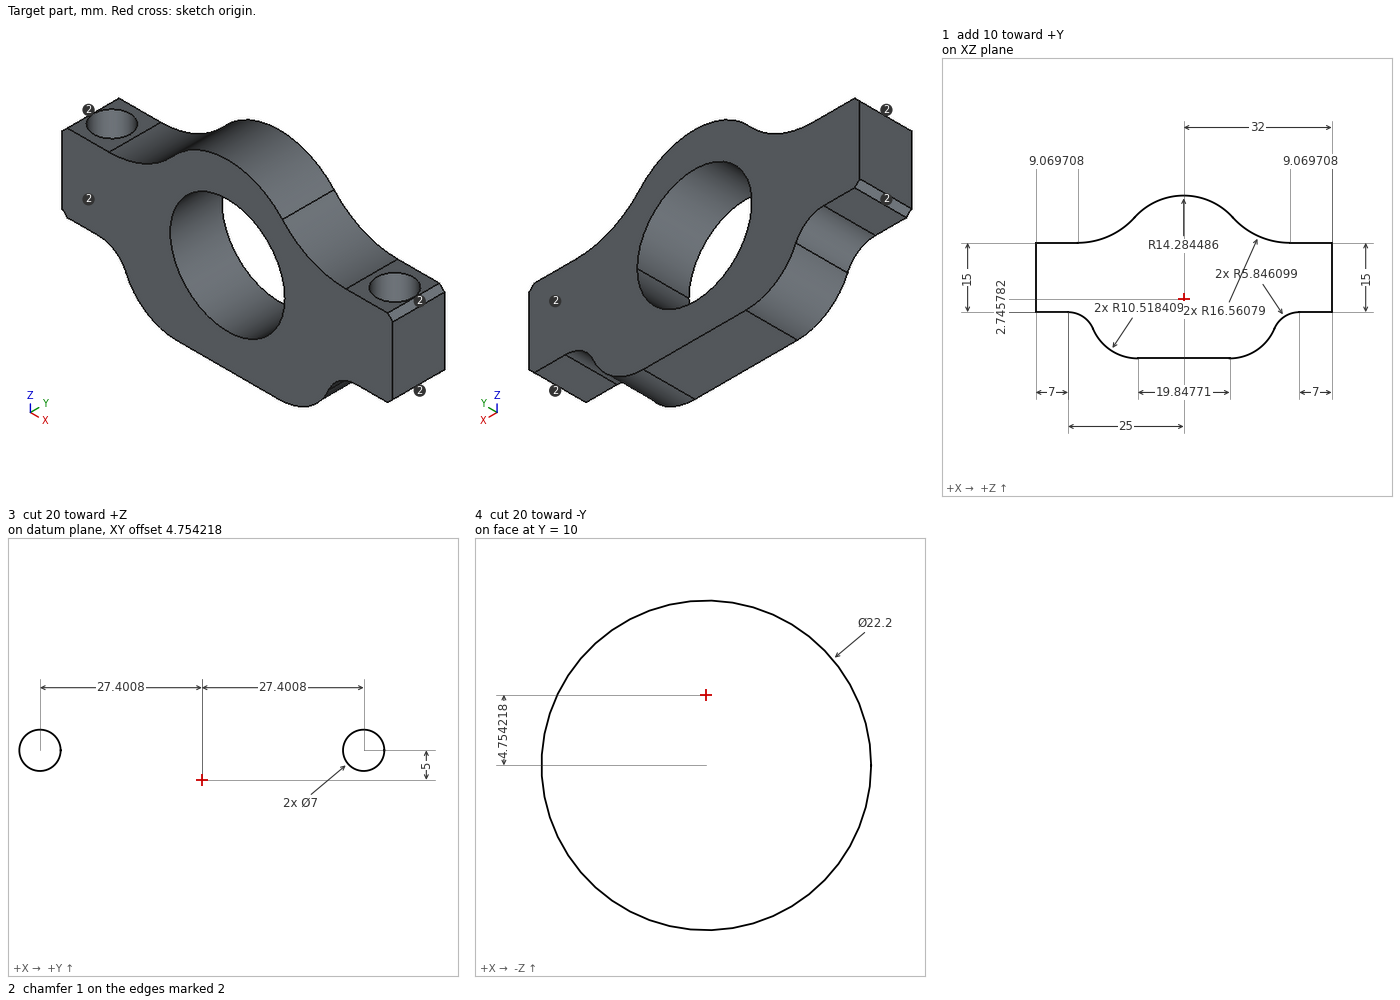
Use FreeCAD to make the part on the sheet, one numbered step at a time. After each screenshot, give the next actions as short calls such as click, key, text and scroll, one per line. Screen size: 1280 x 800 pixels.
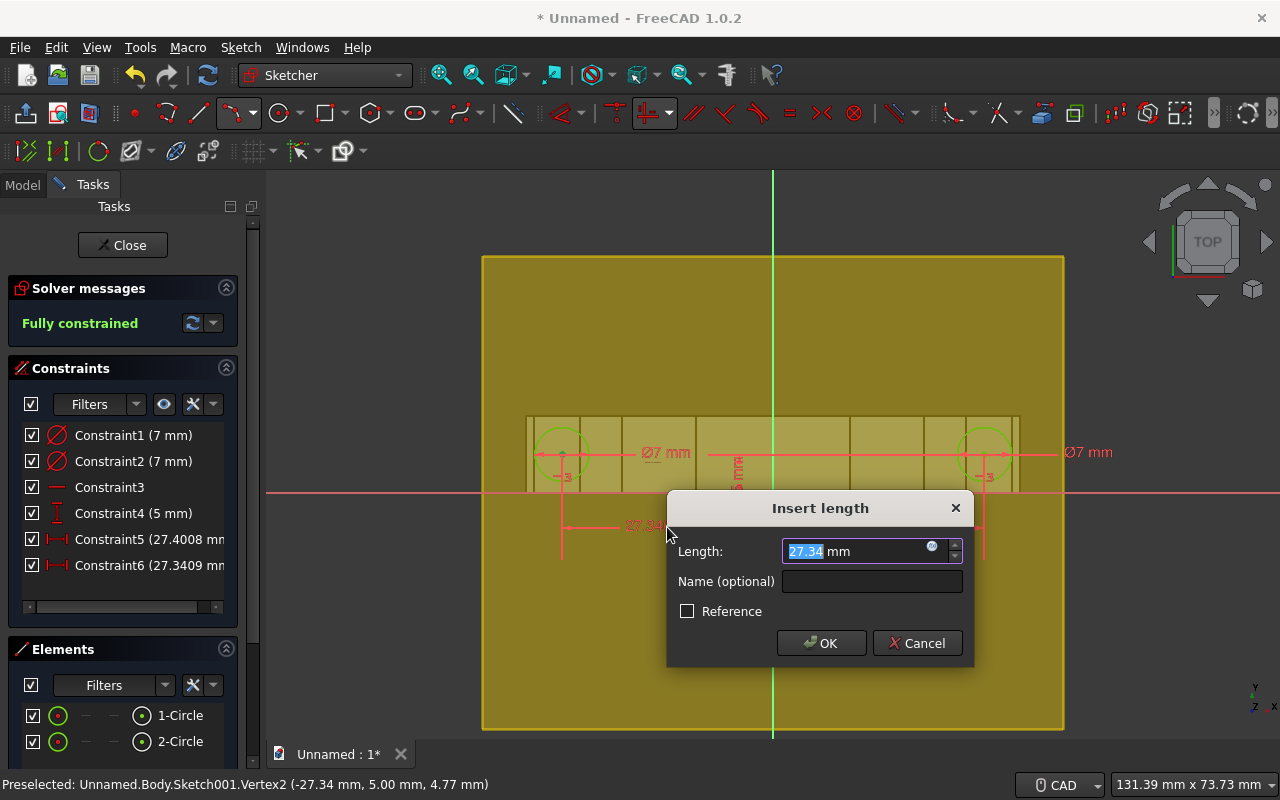
text(27.4008)
key(Return)
key(Escape)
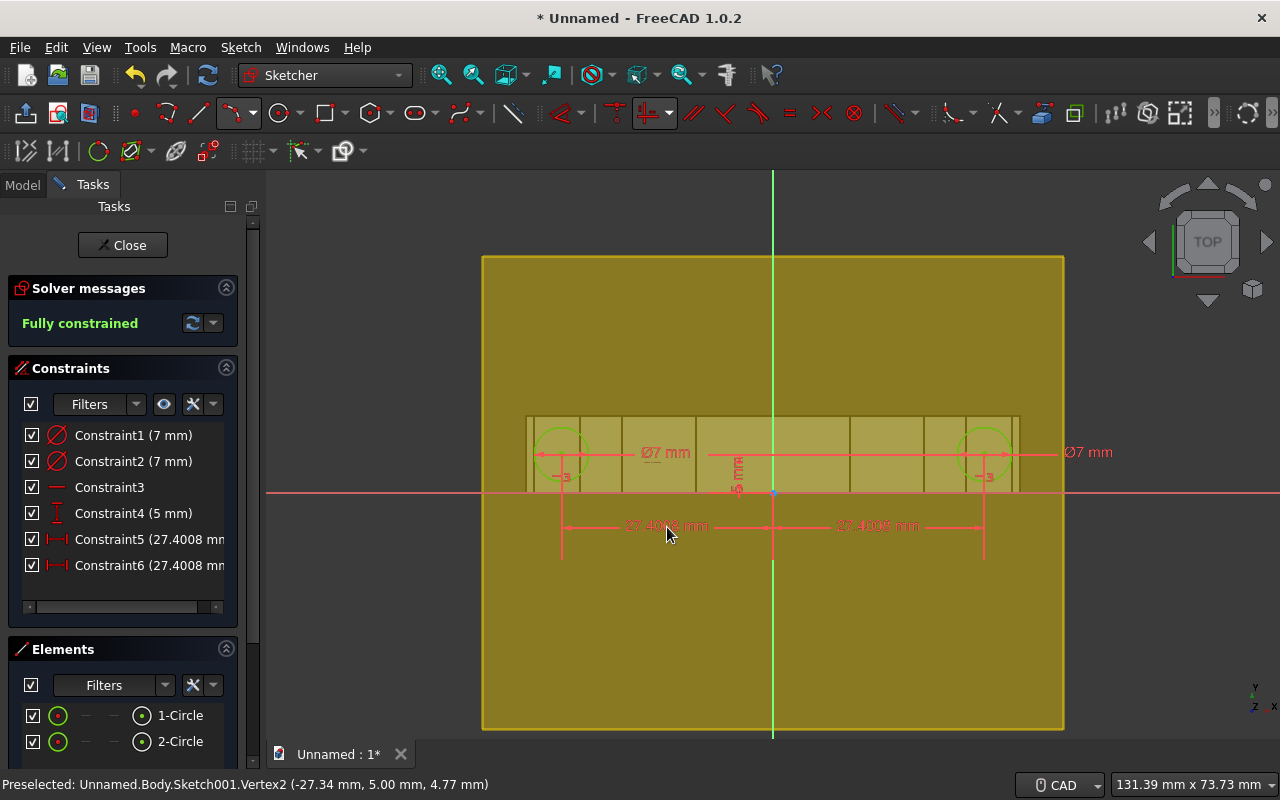
click(123, 245)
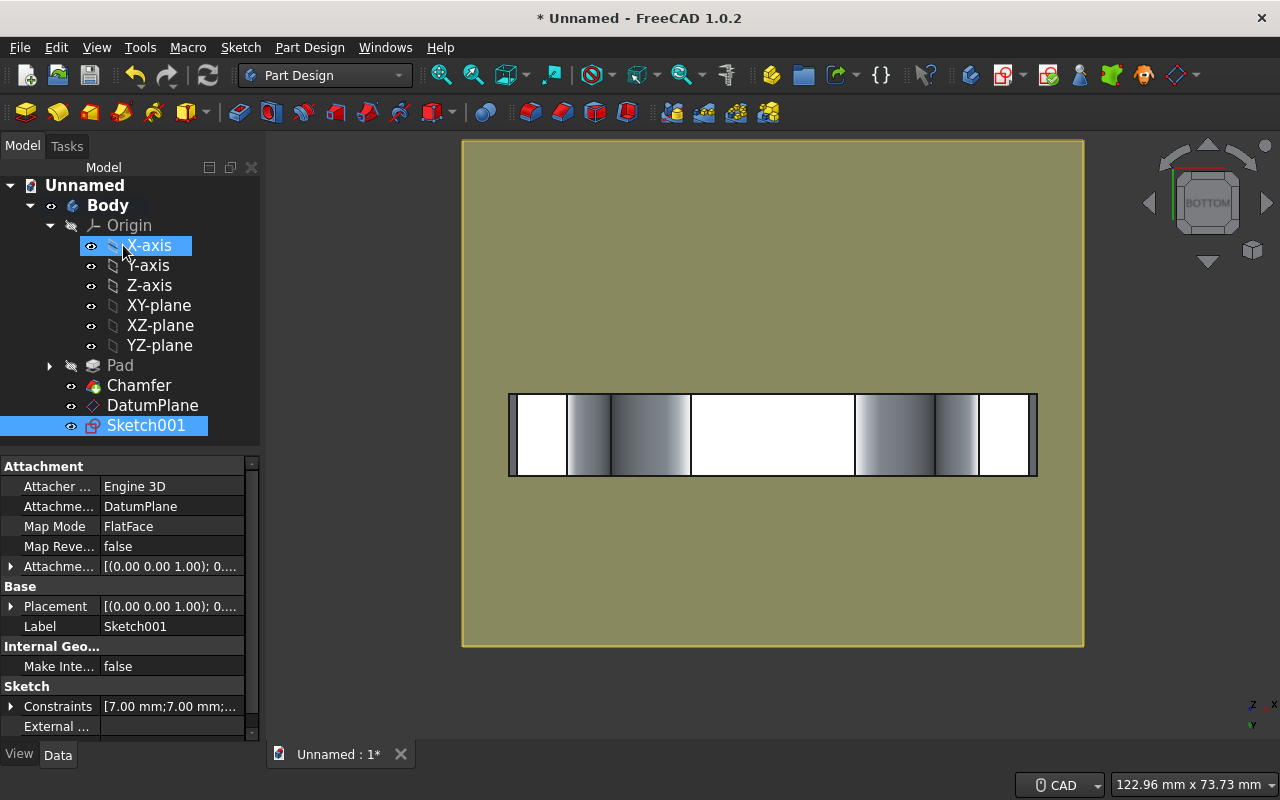
click(240, 112)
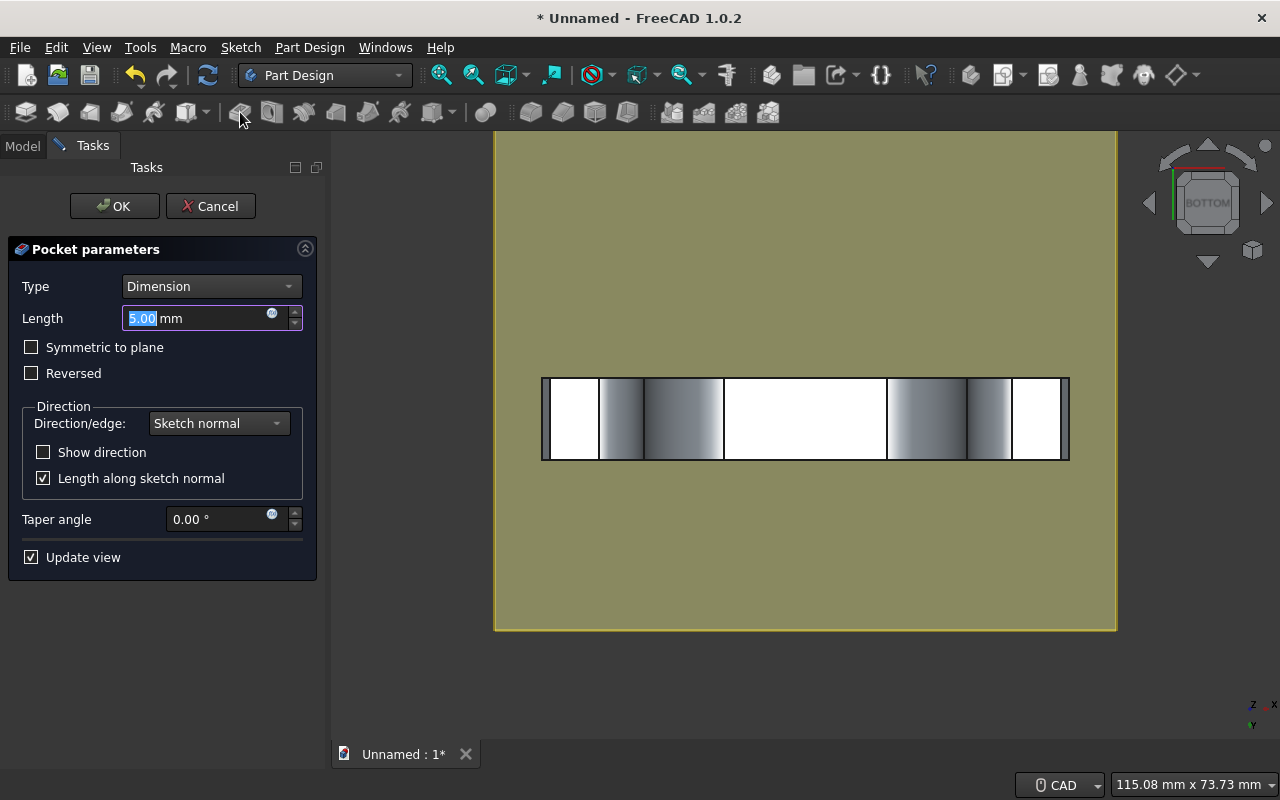
text(20)
key(Tab)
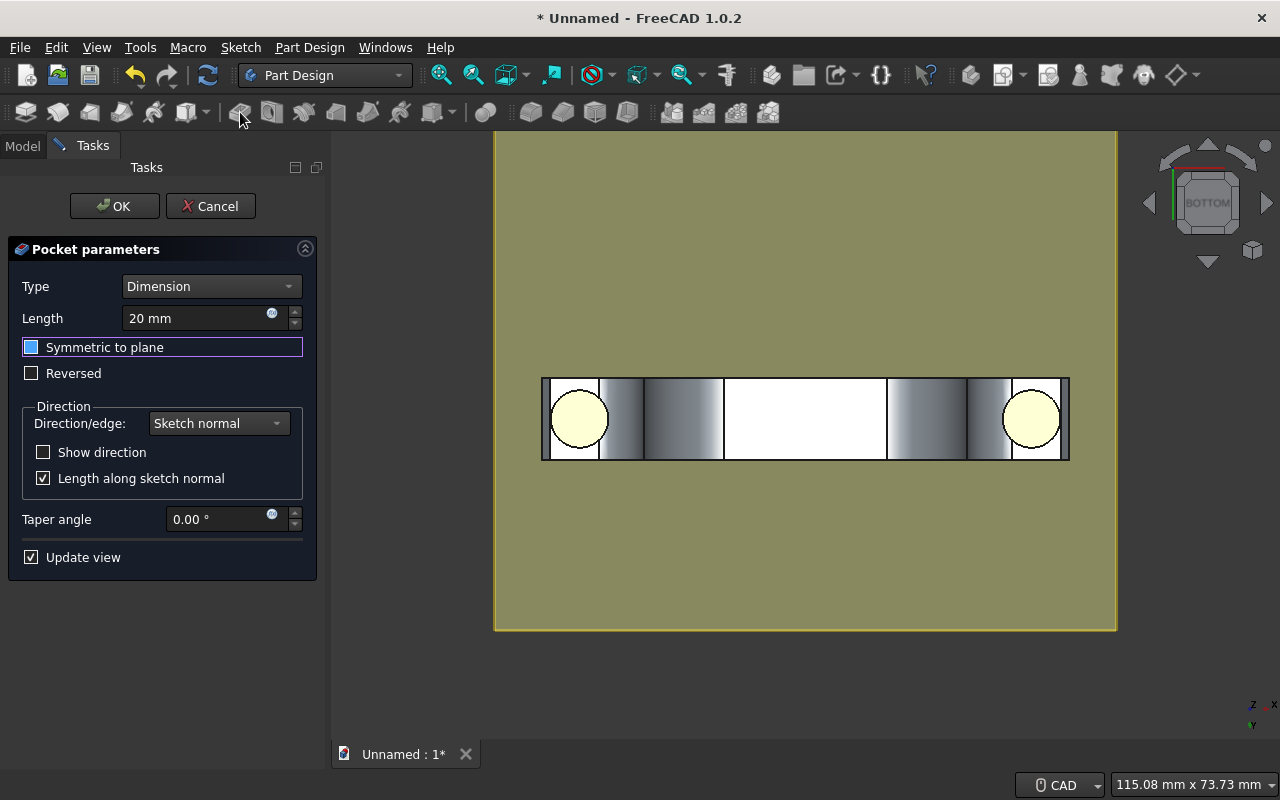
click(30, 373)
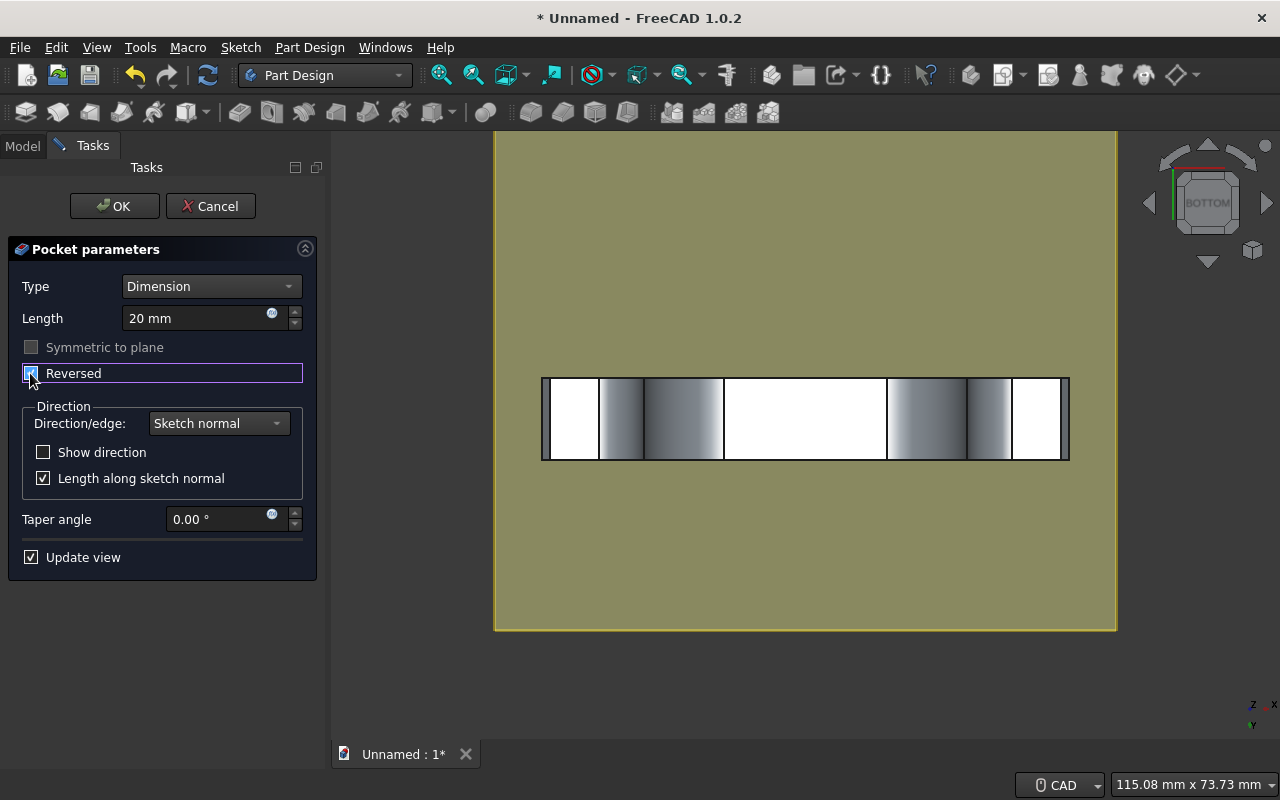
click(115, 206)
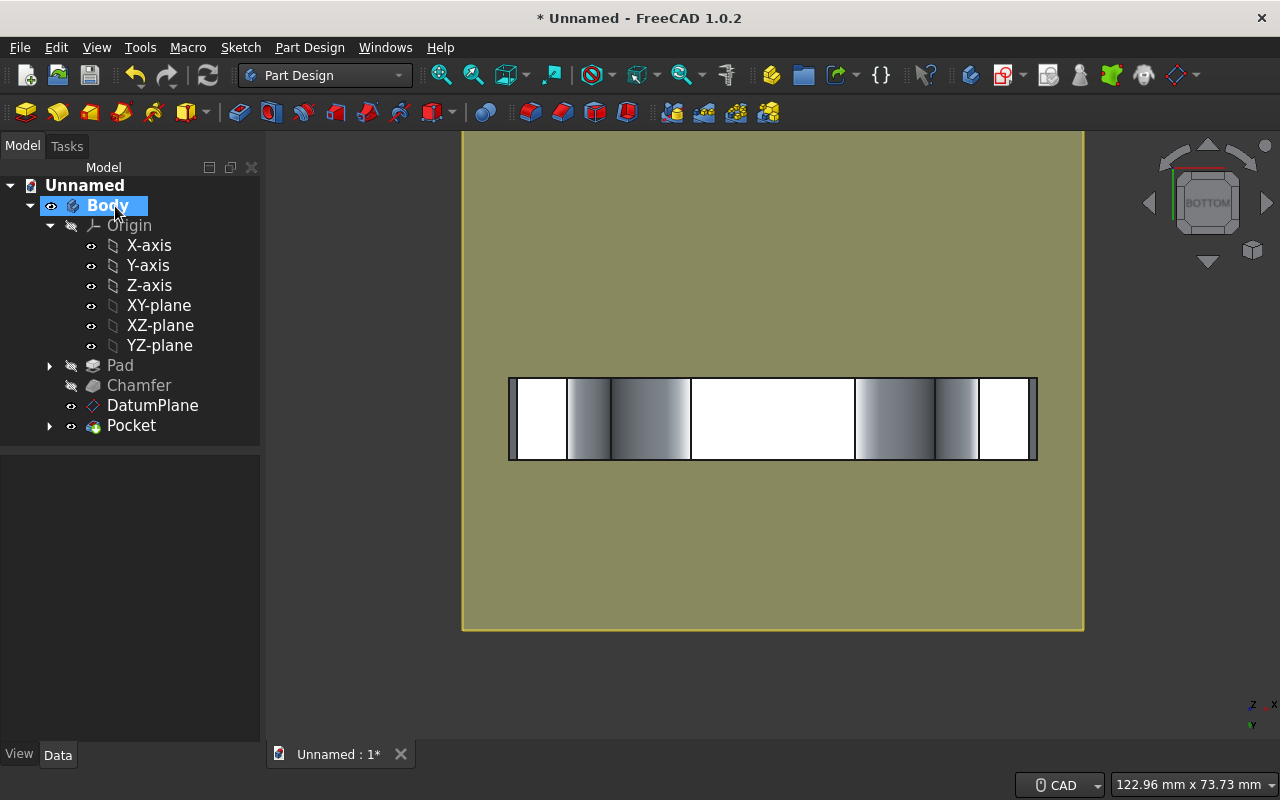
click(116, 406)
key(space)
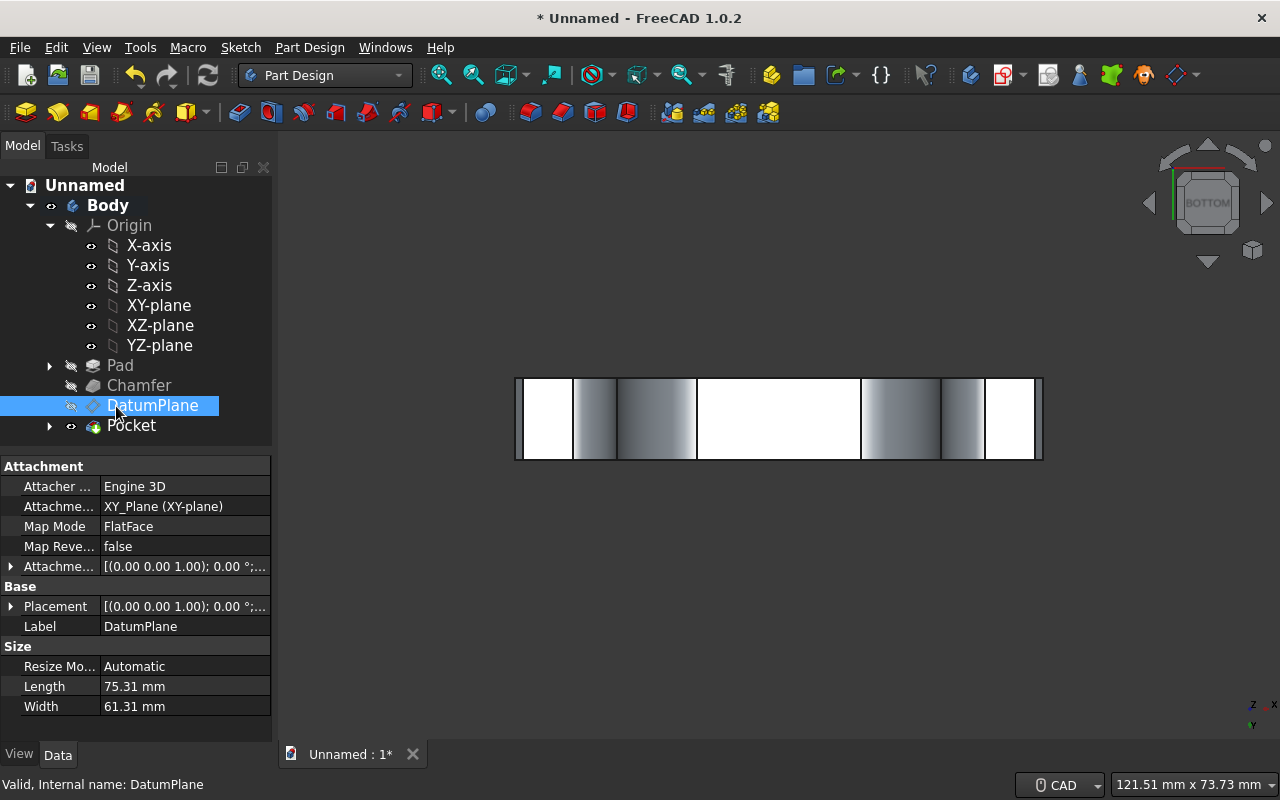
key(4)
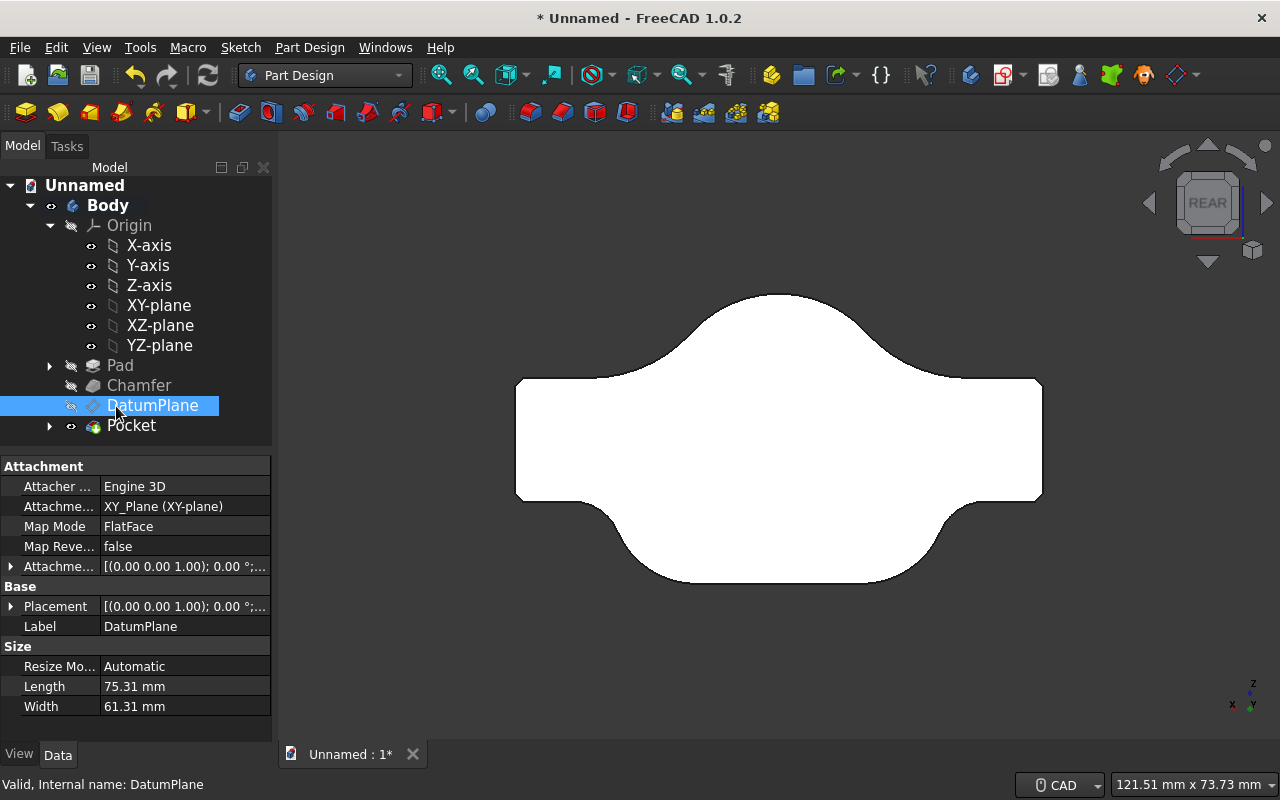
click(779, 438)